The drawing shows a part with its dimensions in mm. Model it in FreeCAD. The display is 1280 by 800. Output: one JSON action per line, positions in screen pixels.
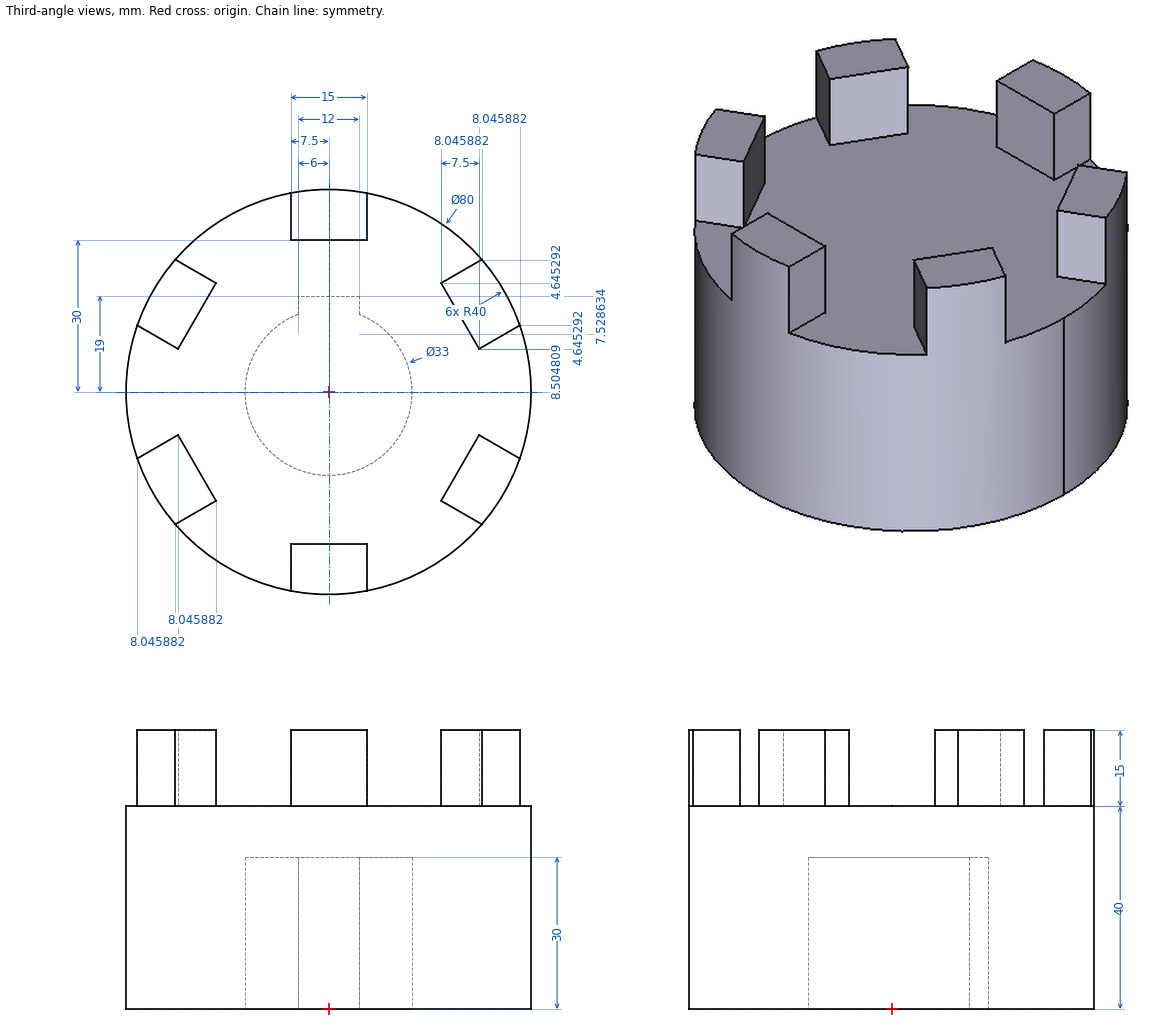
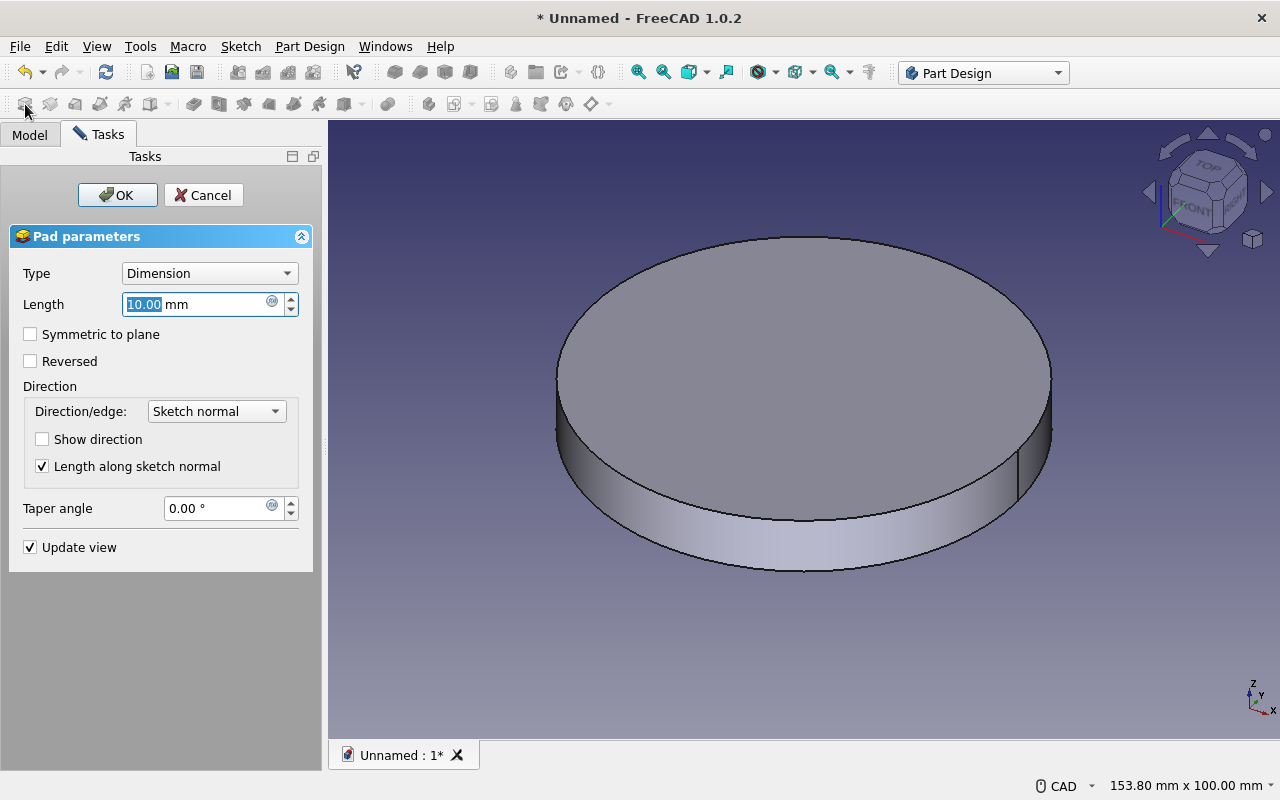
{"action": "type", "text": "40"}
{"action": "key", "text": "Tab"}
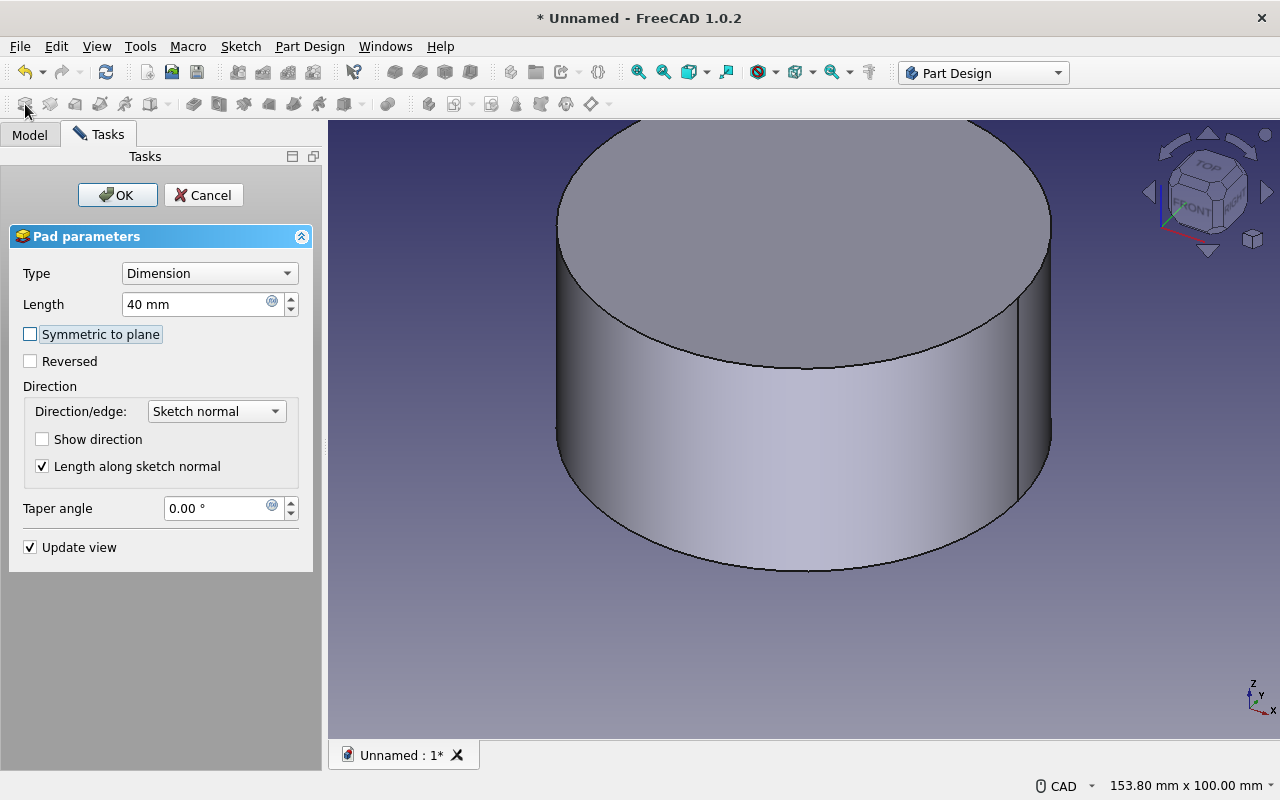
{"action": "left_click", "coordinate": [118, 195]}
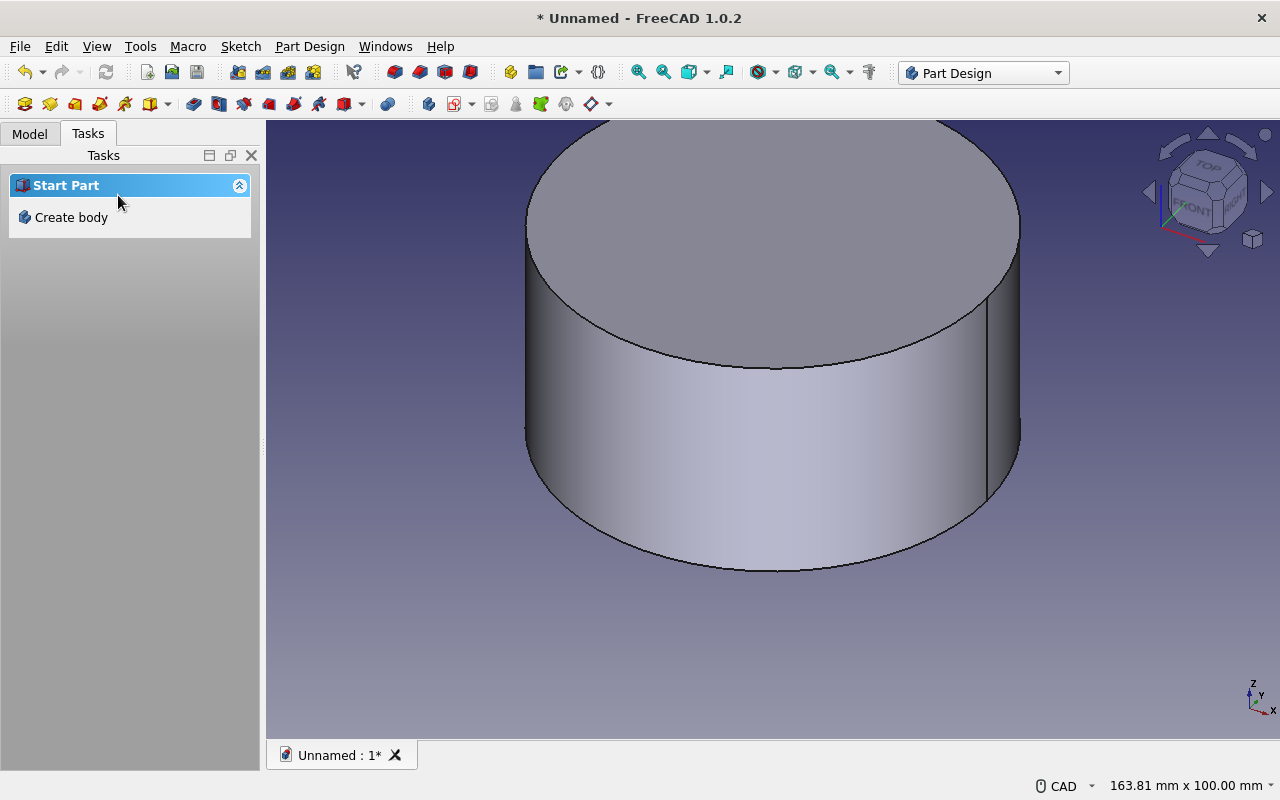
{"action": "key", "text": "v f"}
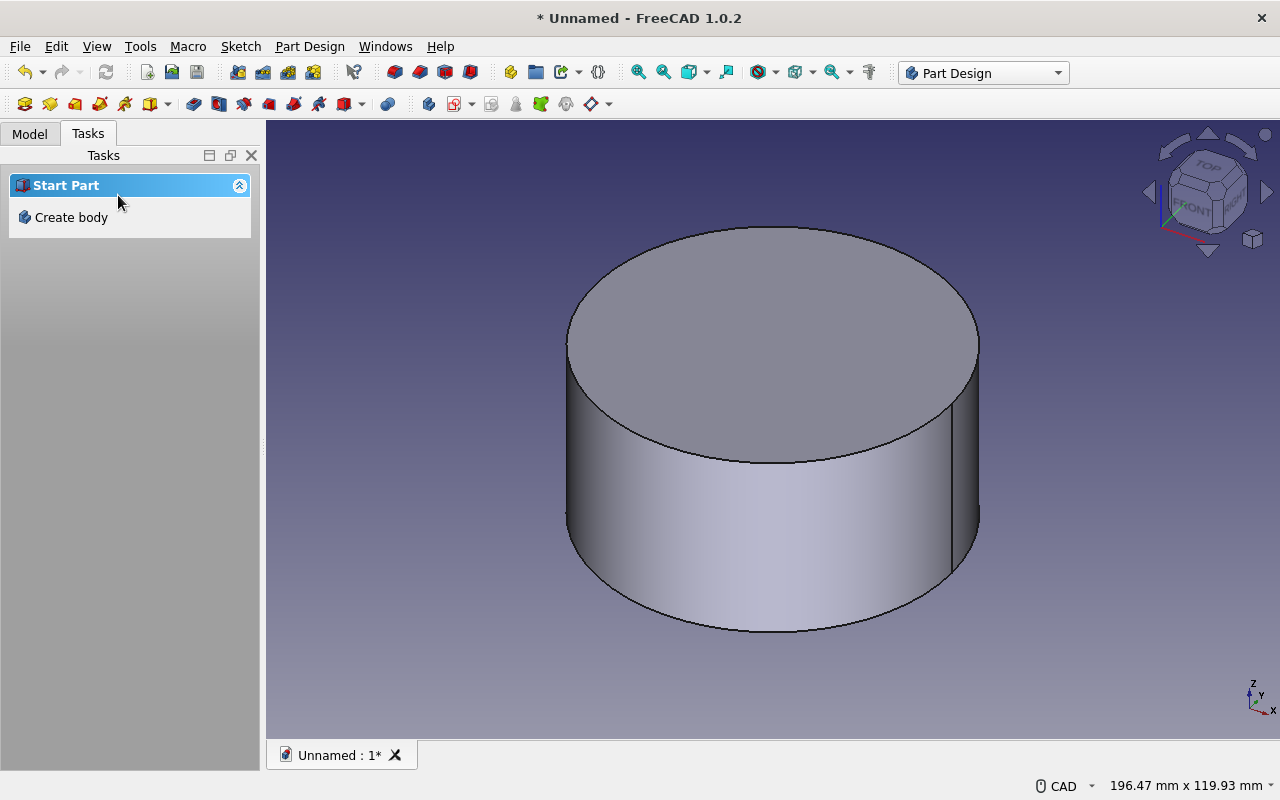
{"action": "key", "text": "5"}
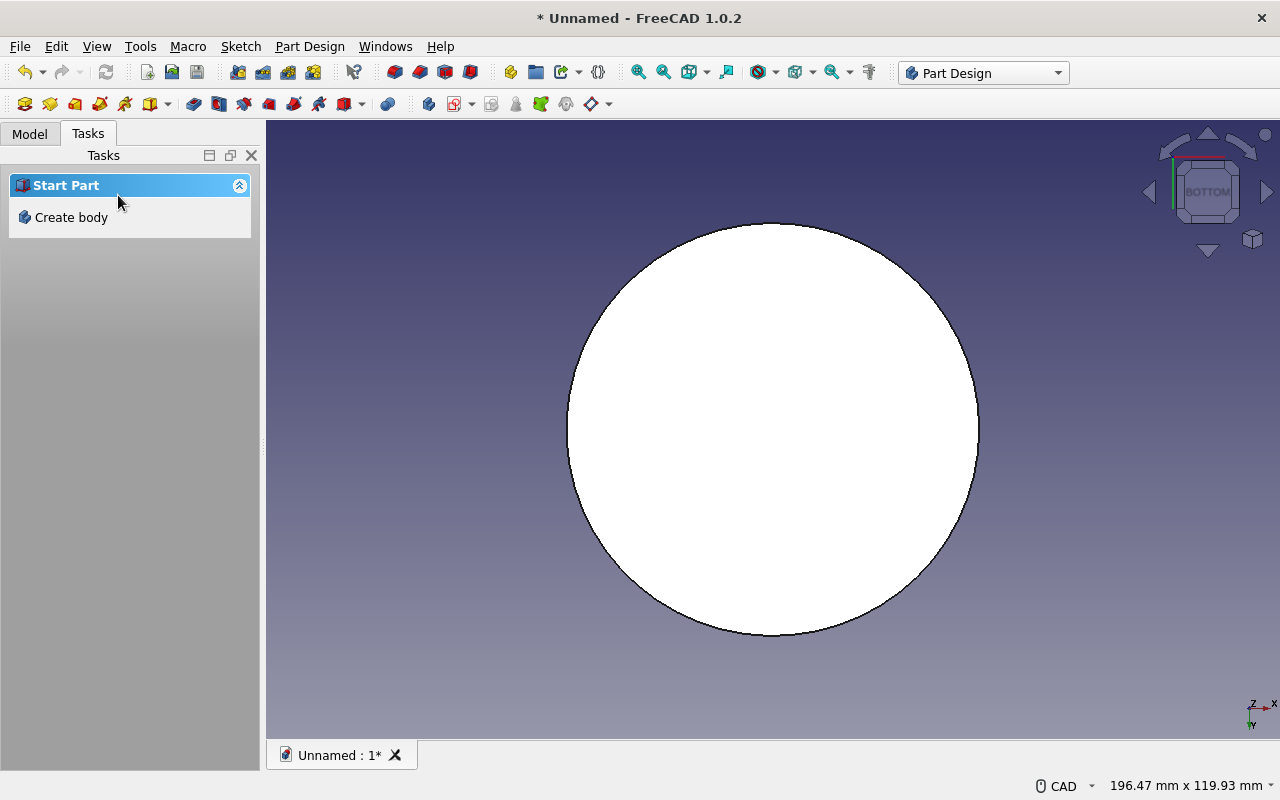
{"action": "left_click", "coordinate": [773, 428]}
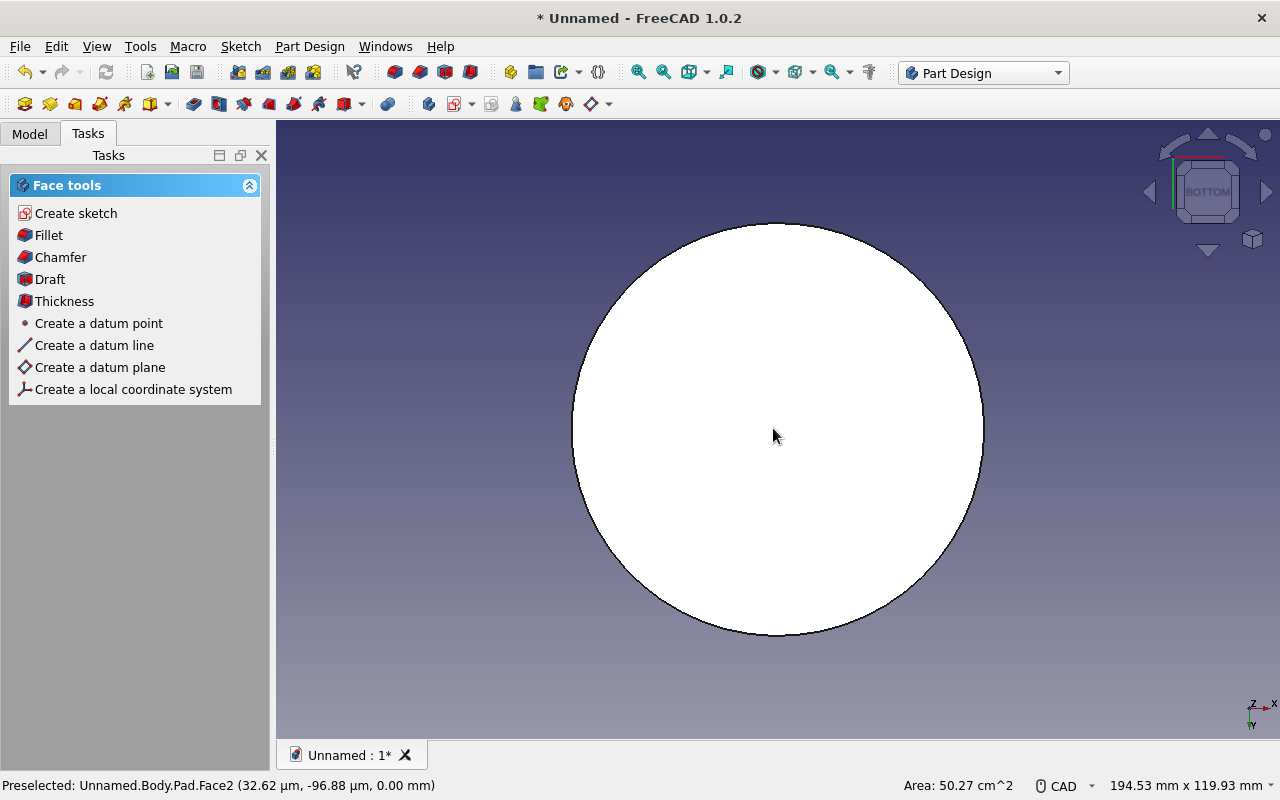
{"action": "left_click", "coordinate": [454, 104]}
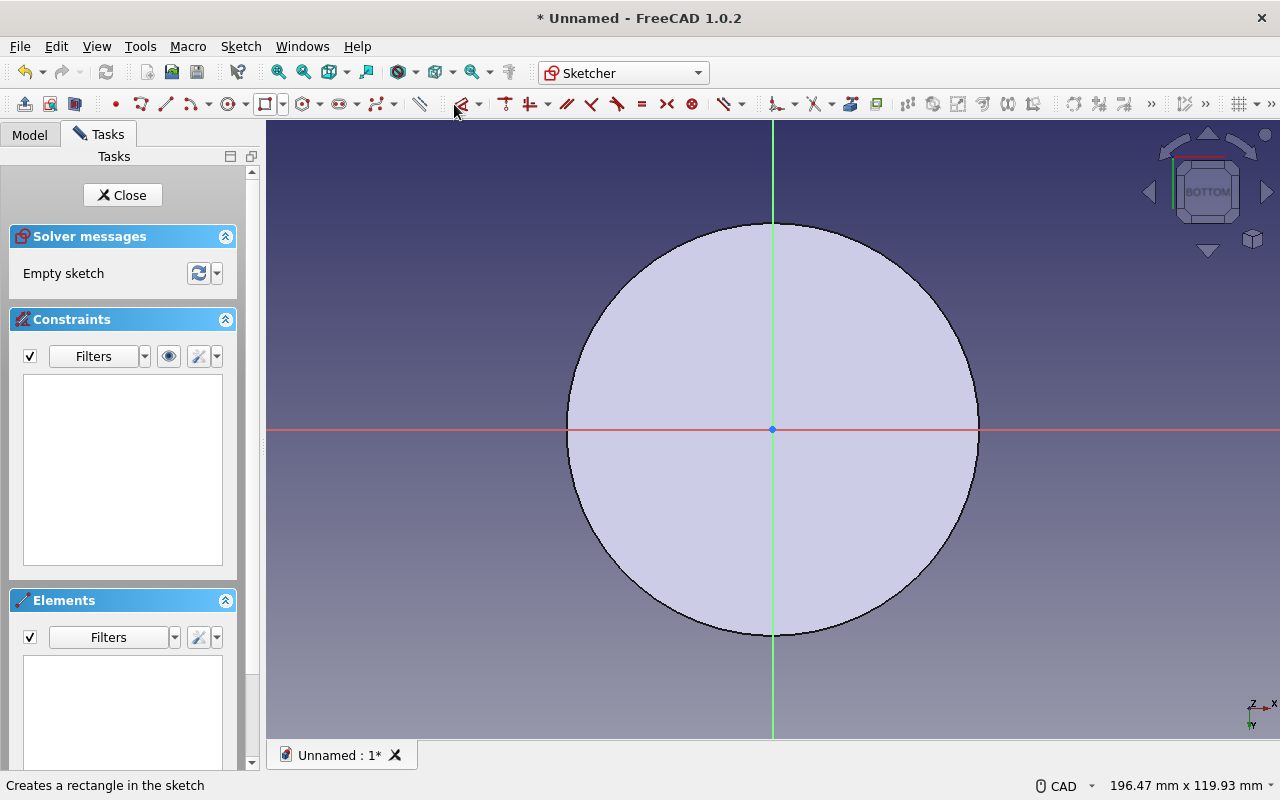
{"action": "scroll", "coordinate": [829, 430], "scroll_direction": "up", "scroll_amount": 4}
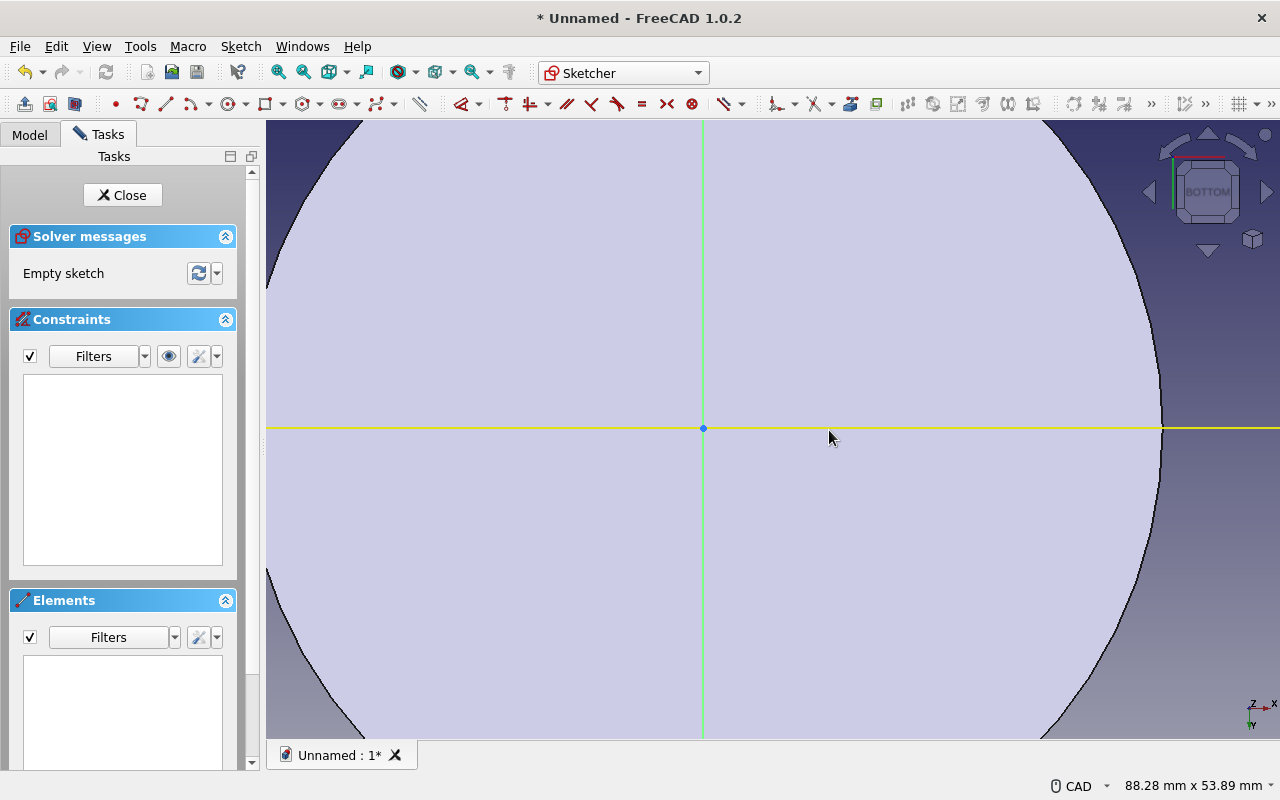
{"action": "key", "text": "g c"}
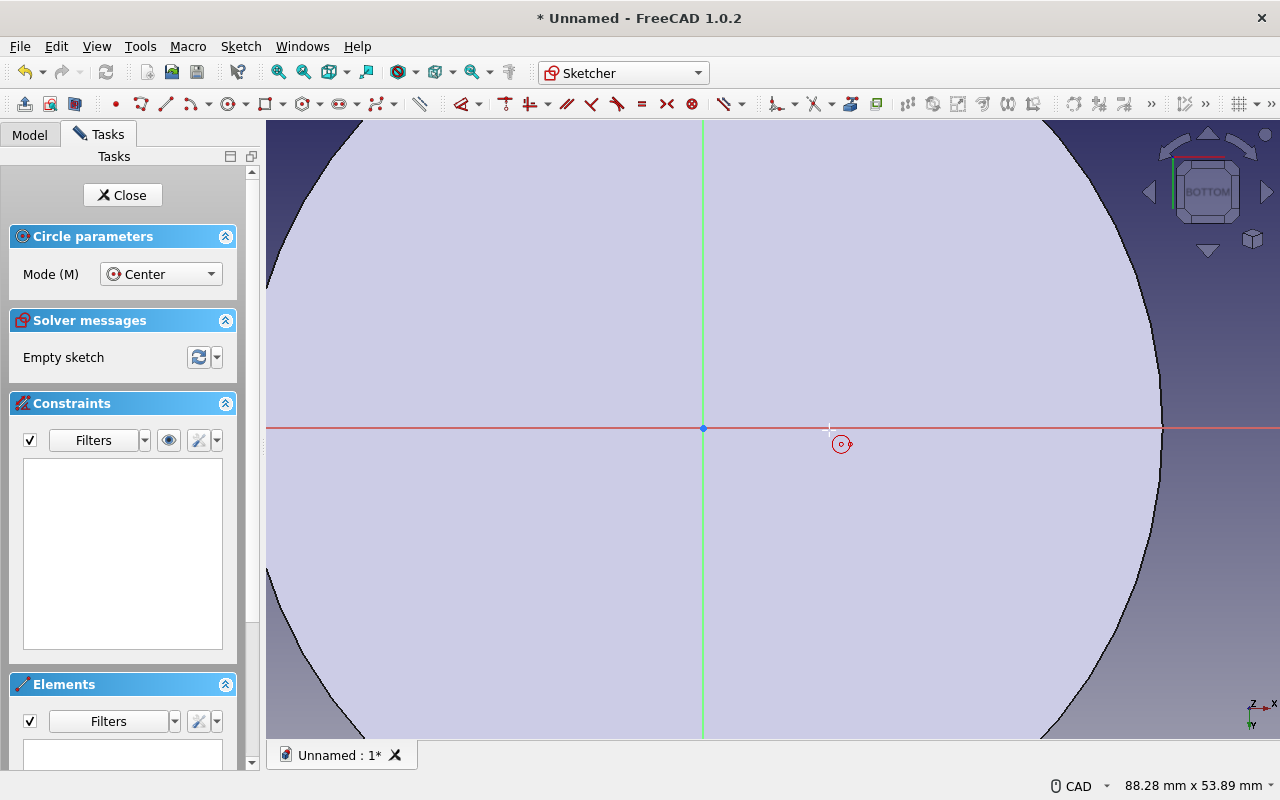
{"action": "left_click", "coordinate": [703, 428]}
{"action": "mouse_move", "coordinate": [837, 294]}